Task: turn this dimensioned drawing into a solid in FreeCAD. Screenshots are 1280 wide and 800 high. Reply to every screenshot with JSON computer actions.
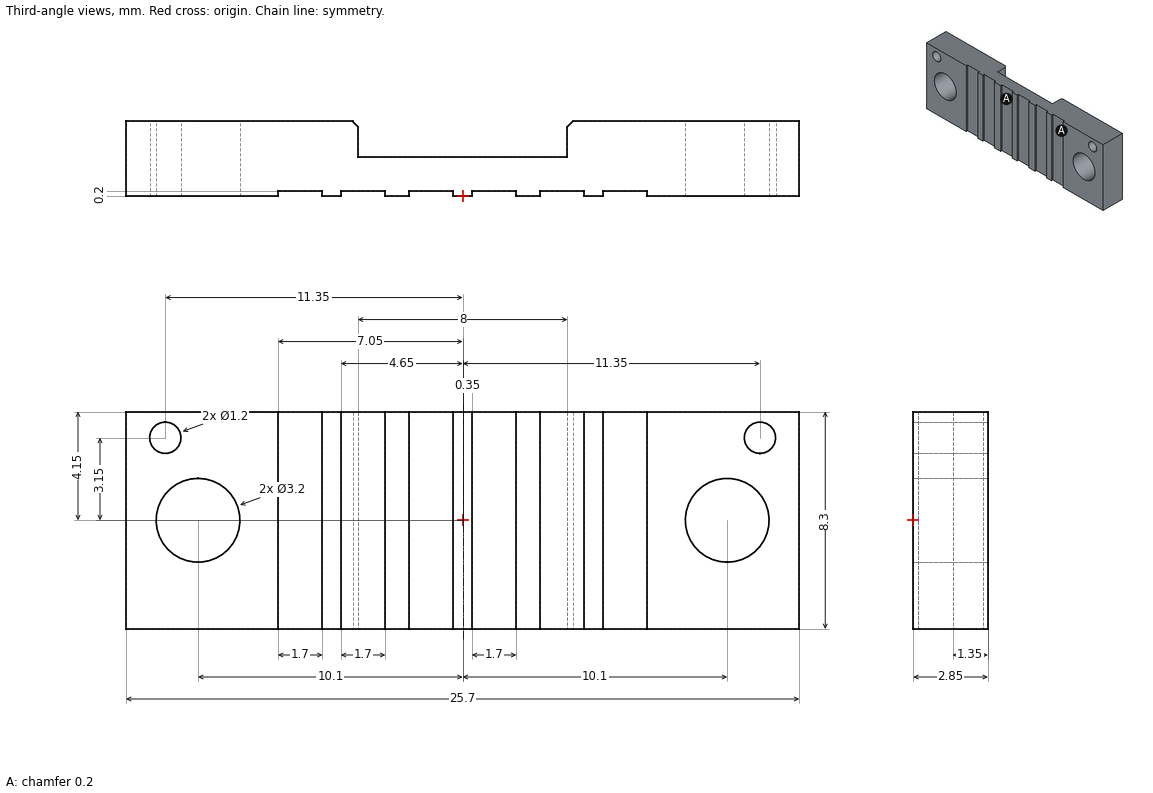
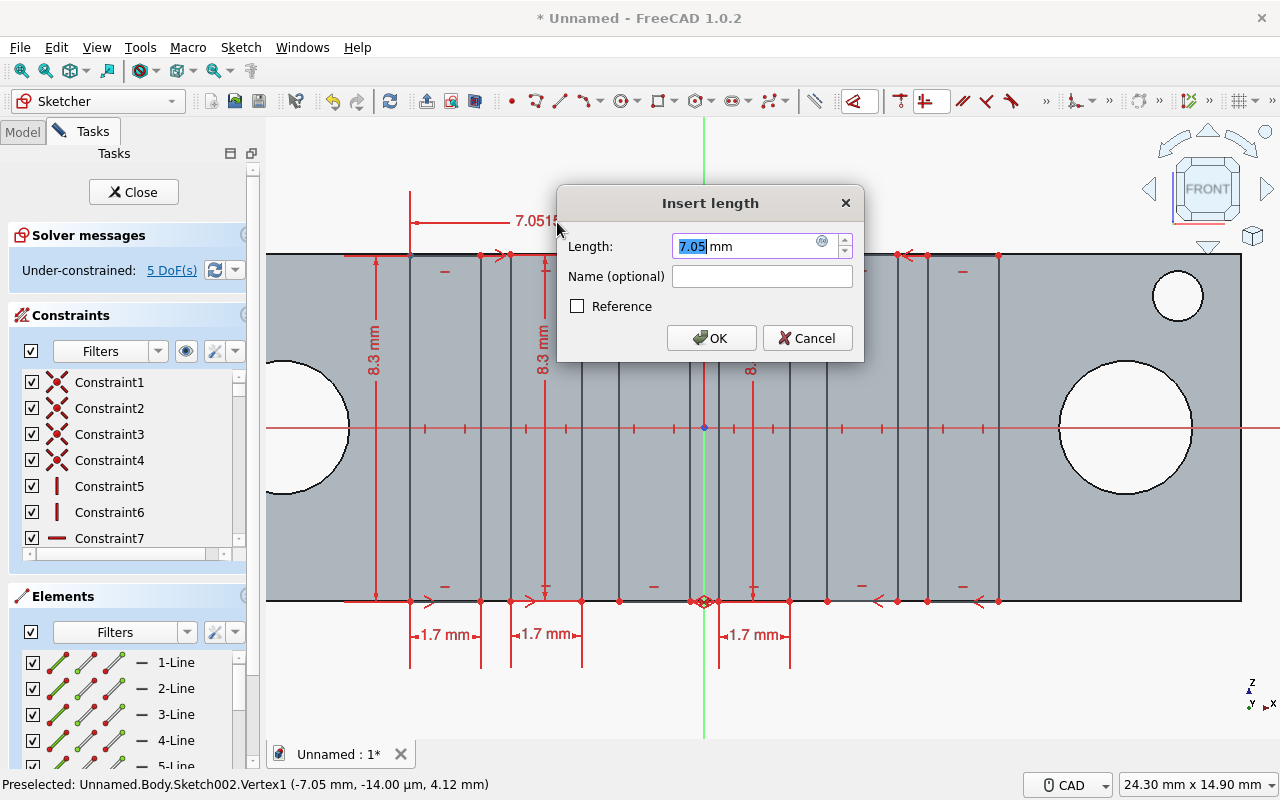
{"action": "type", "text": "7.05"}
{"action": "key", "text": "Return"}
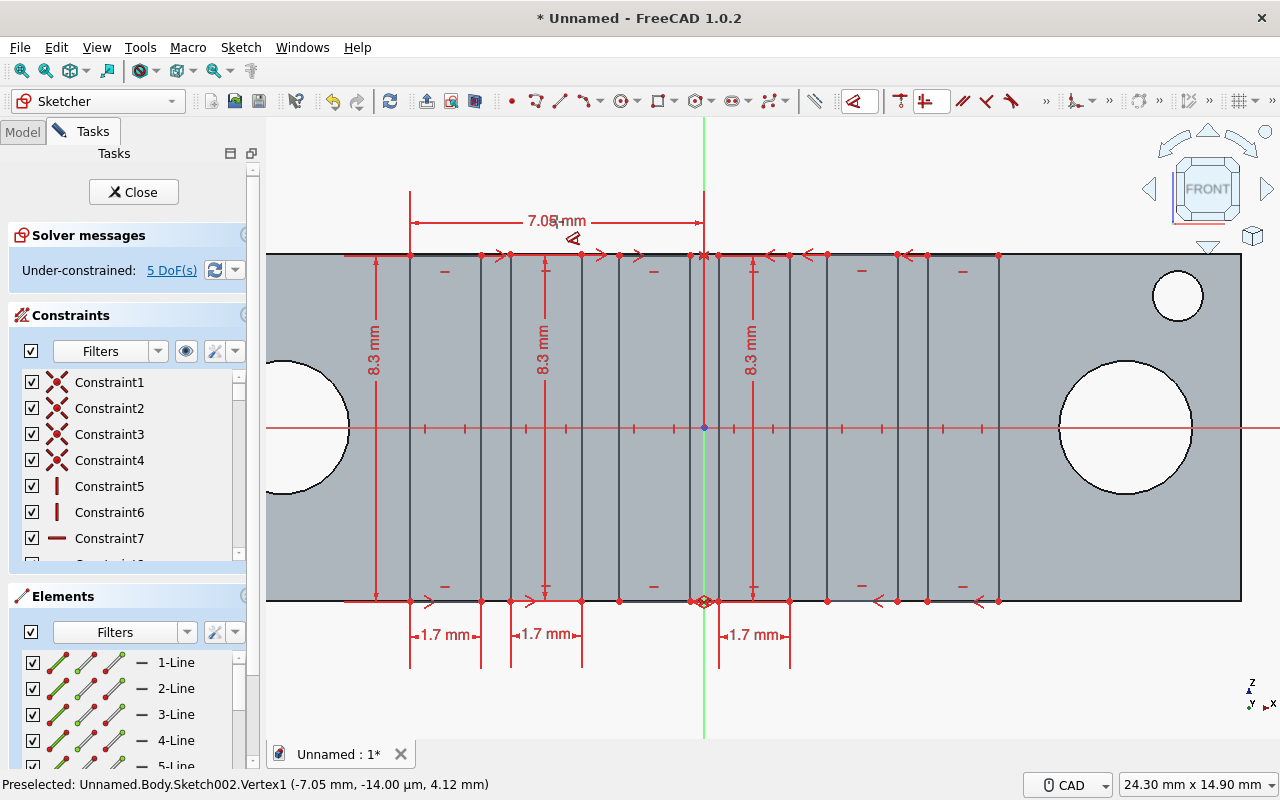
{"action": "left_click", "coordinate": [410, 256]}
{"action": "left_click", "coordinate": [376, 302]}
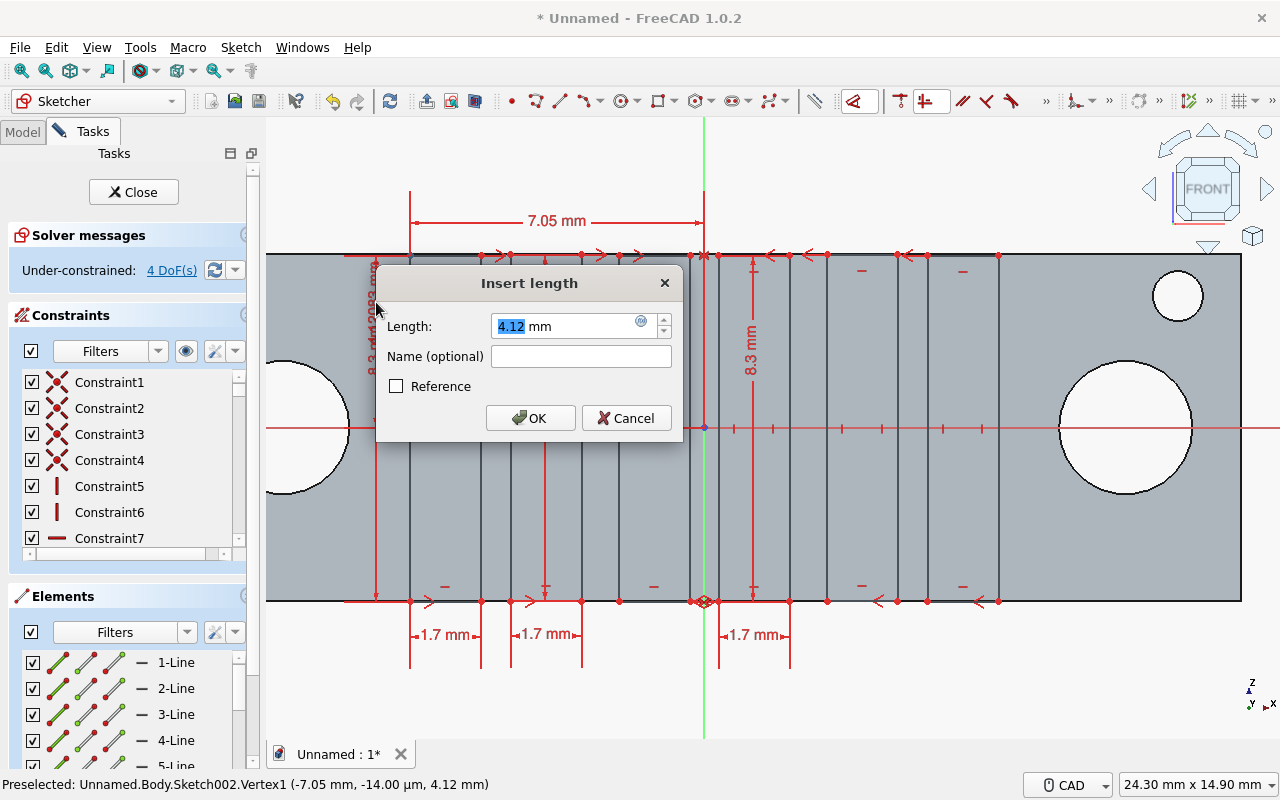
{"action": "type", "text": "4.15"}
{"action": "key", "text": "Return"}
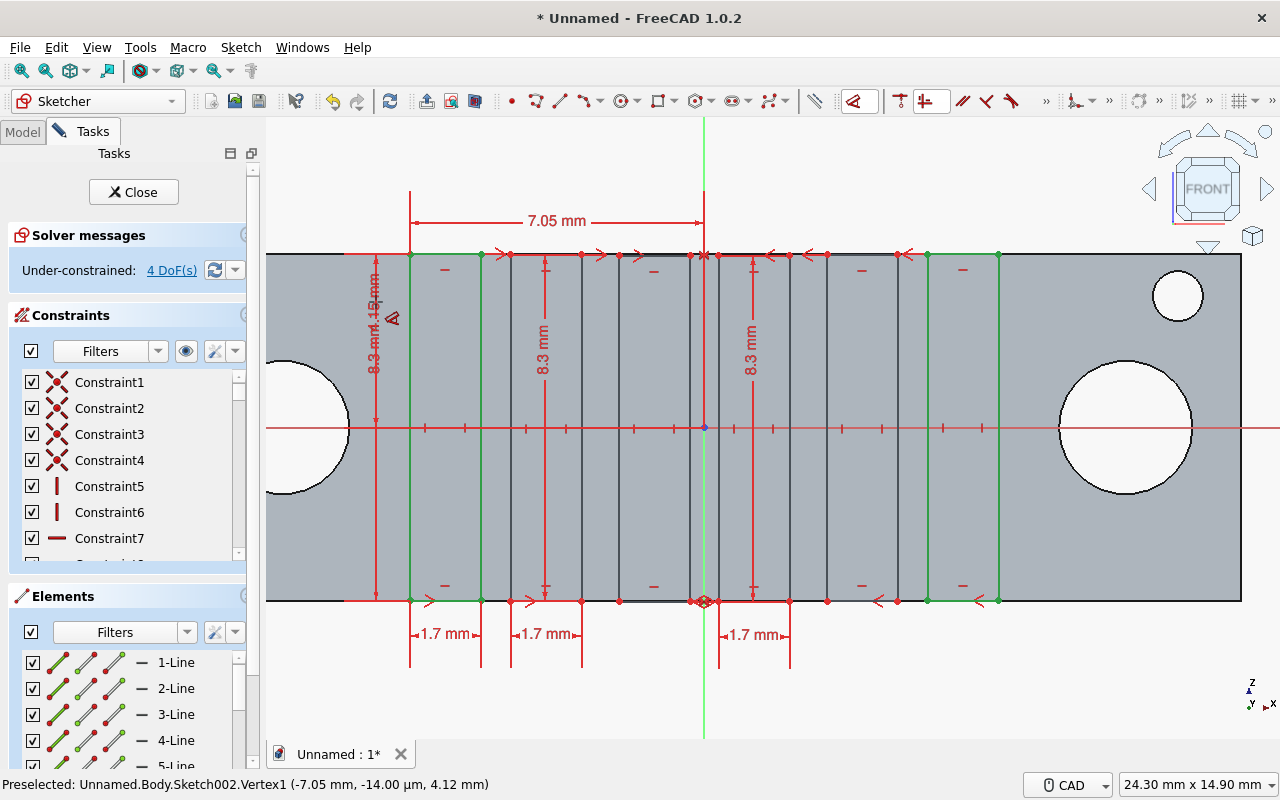
{"action": "scroll", "coordinate": [719, 256], "scroll_direction": "up", "scroll_amount": 5}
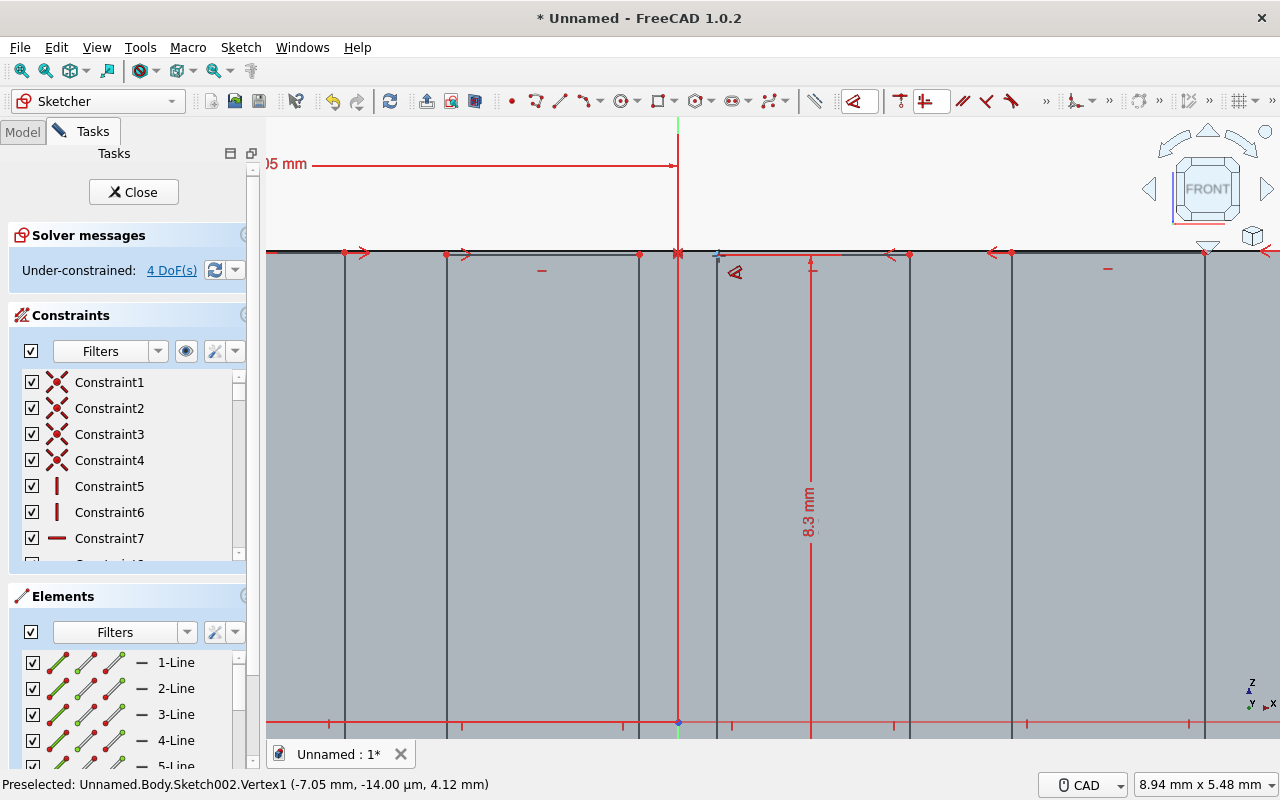
{"action": "left_click", "coordinate": [717, 255]}
{"action": "left_click", "coordinate": [698, 221]}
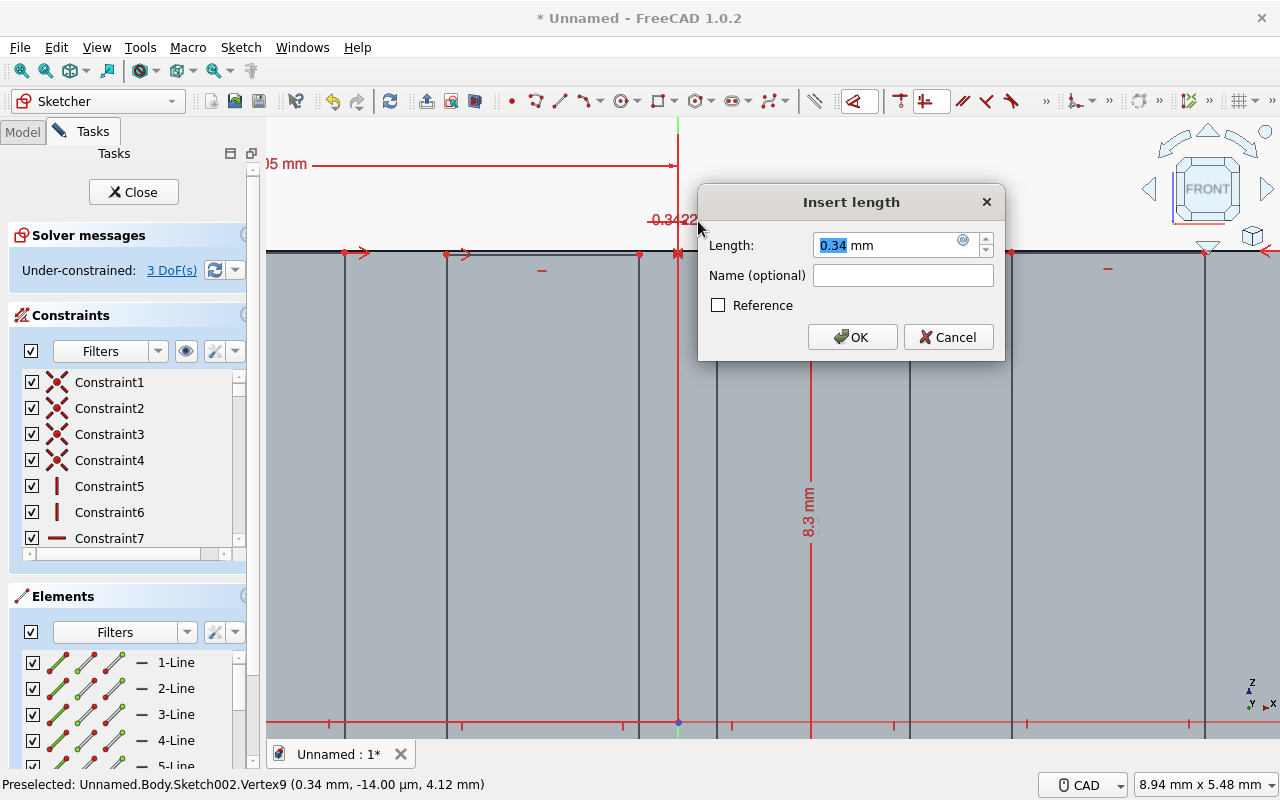
{"action": "type", "text": "0.35"}
{"action": "key", "text": "Return"}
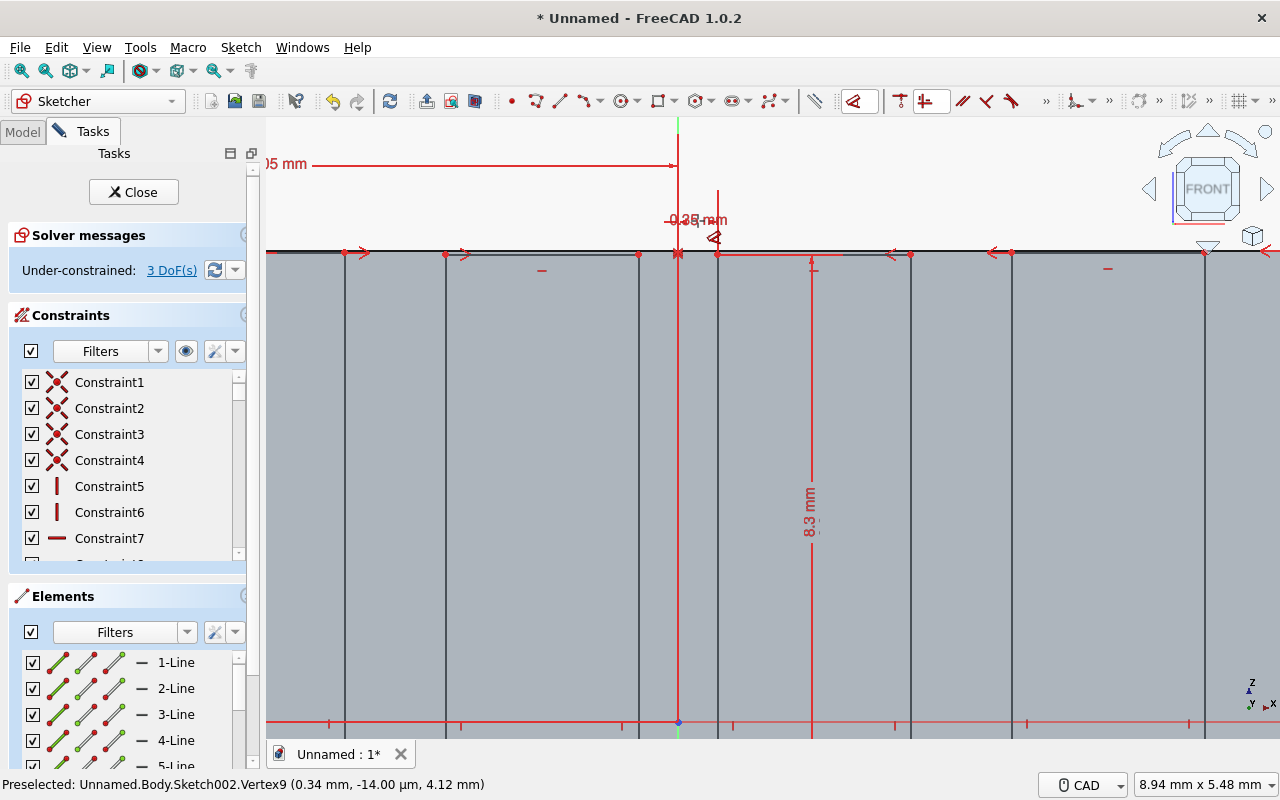
{"action": "left_click", "coordinate": [718, 255]}
{"action": "left_click", "coordinate": [752, 483]}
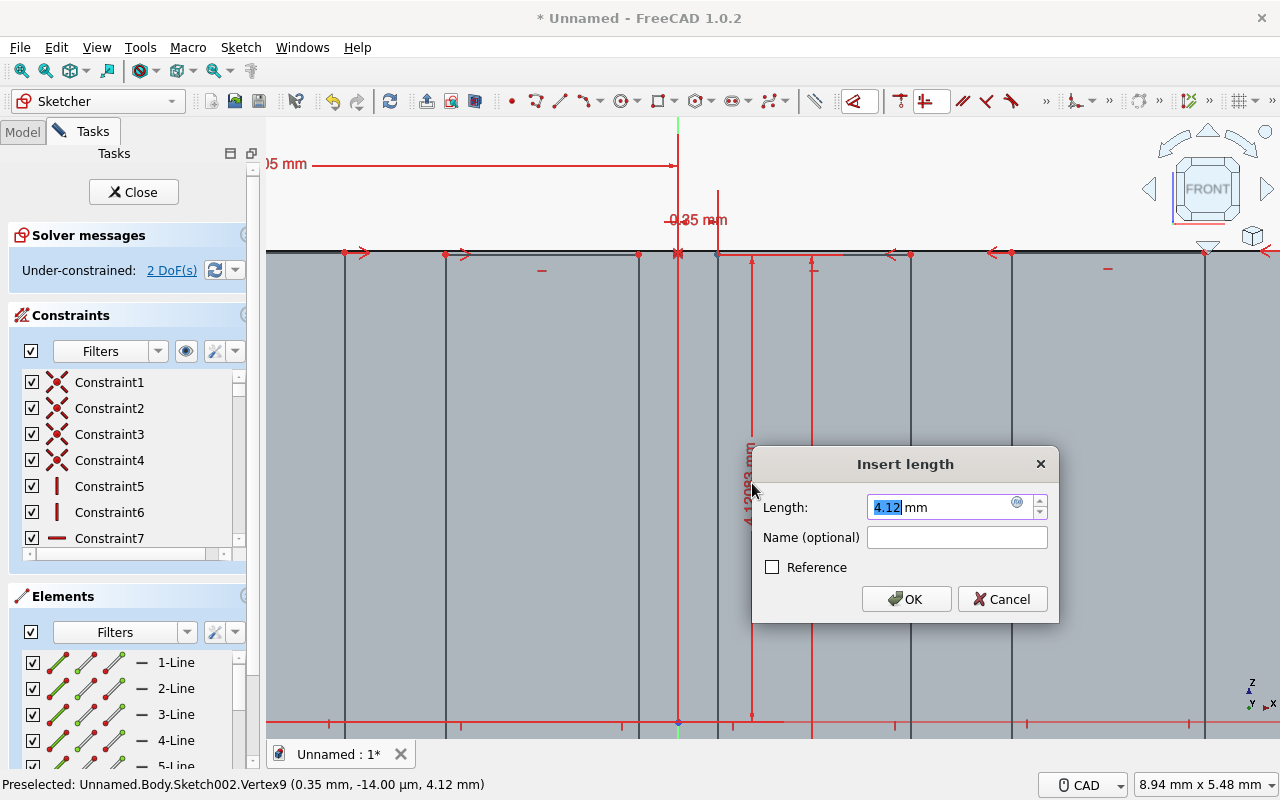
{"action": "type", "text": "4.15"}
{"action": "key", "text": "Return"}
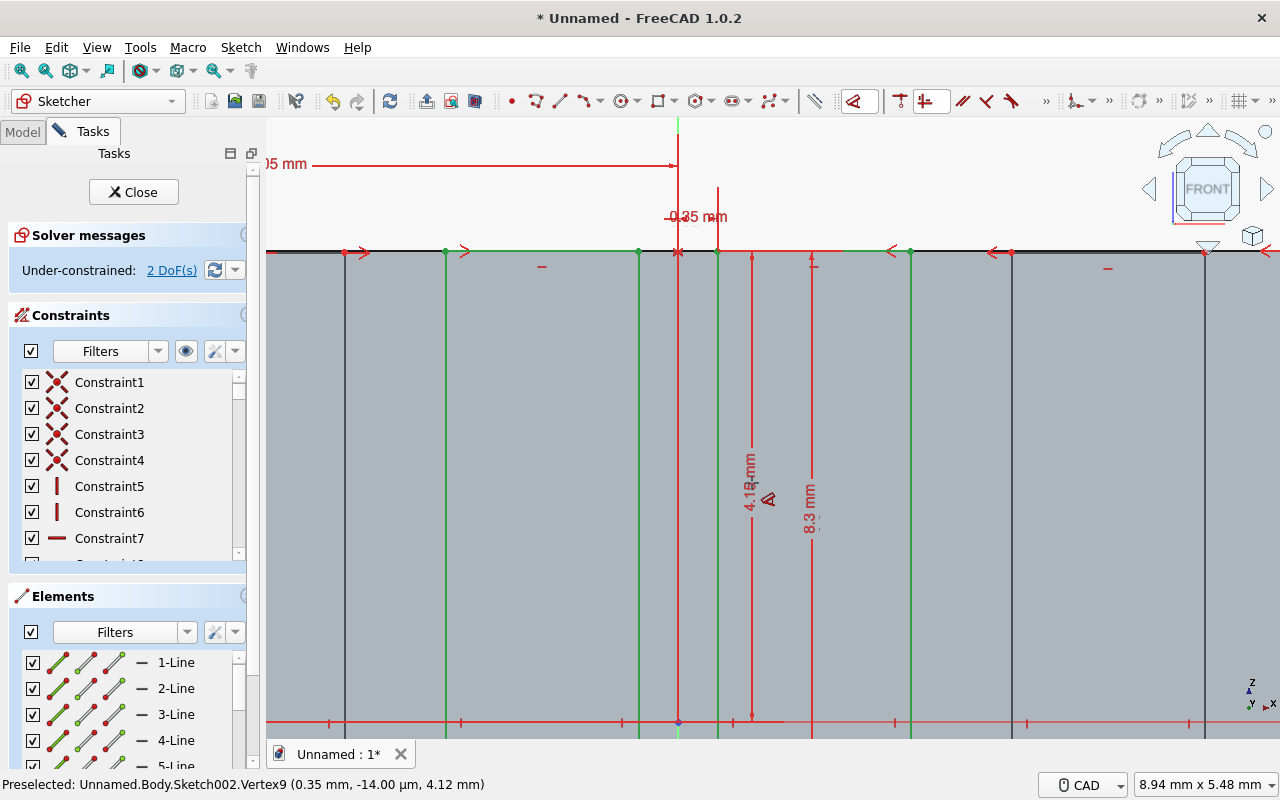
{"action": "scroll", "coordinate": [720, 257], "scroll_direction": "down", "scroll_amount": 5}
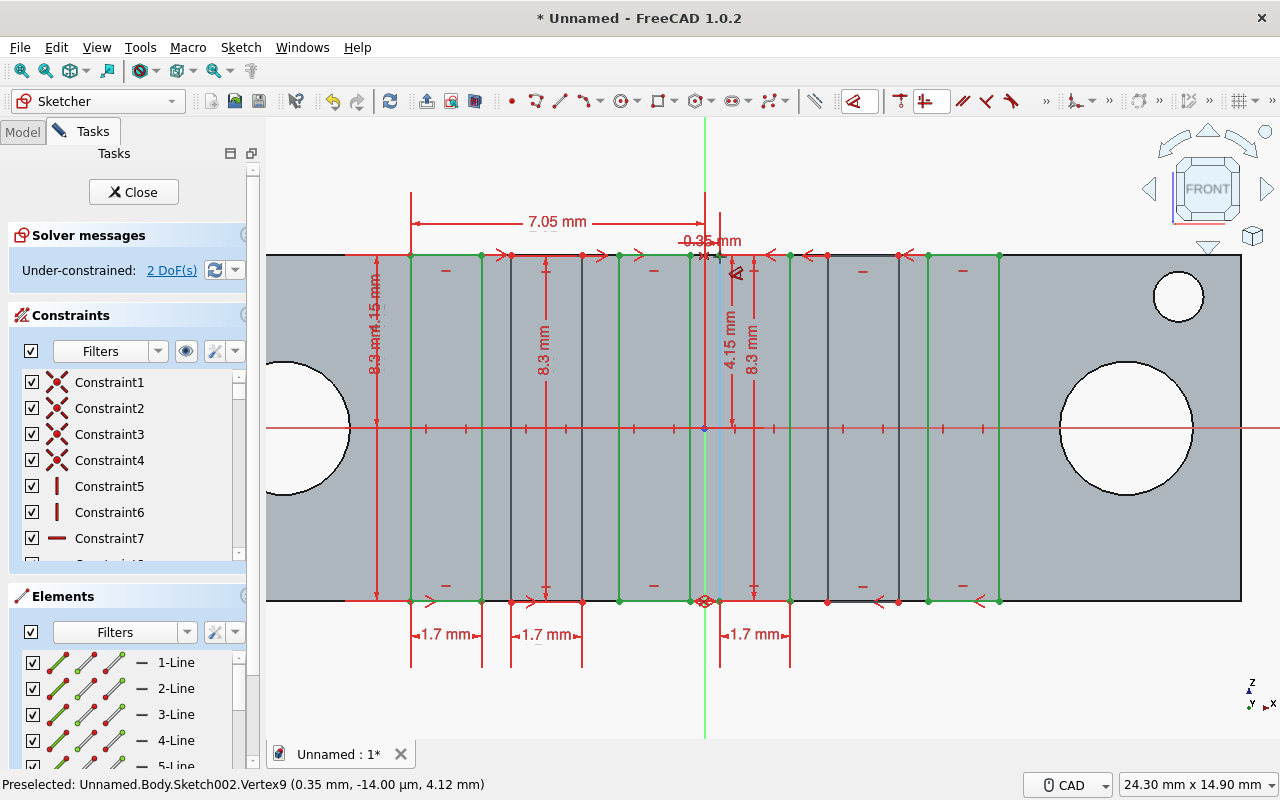
{"action": "left_click", "coordinate": [511, 256]}
{"action": "left_click", "coordinate": [653, 222]}